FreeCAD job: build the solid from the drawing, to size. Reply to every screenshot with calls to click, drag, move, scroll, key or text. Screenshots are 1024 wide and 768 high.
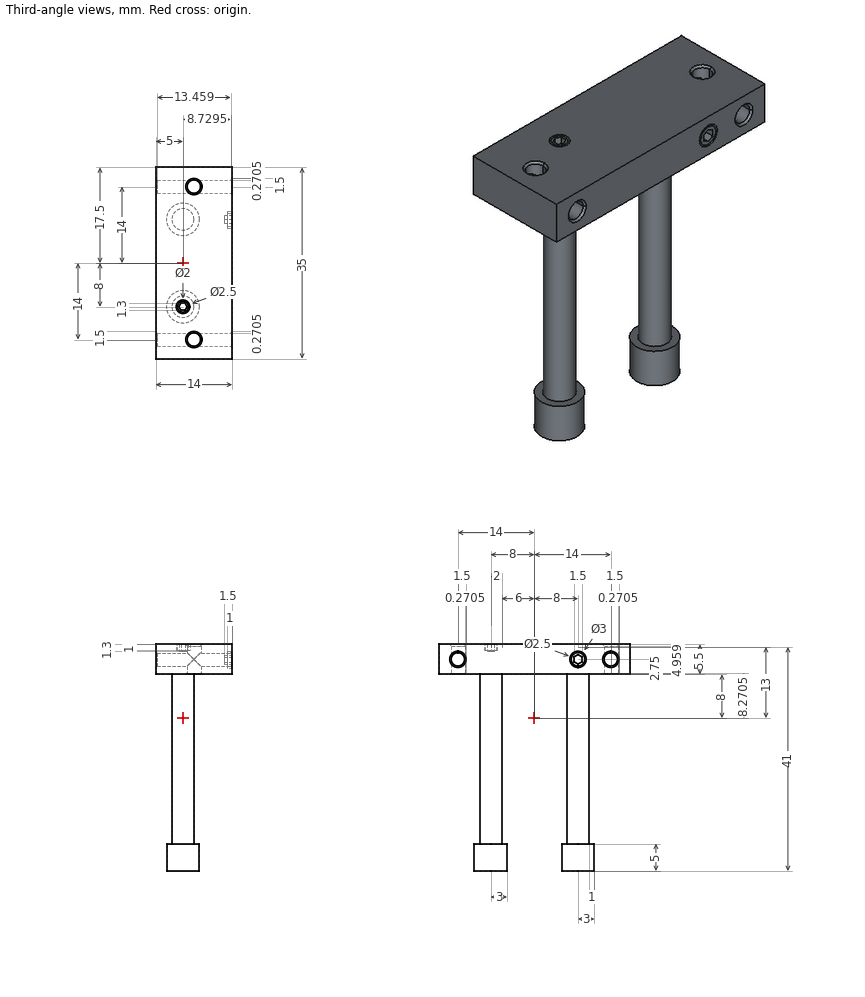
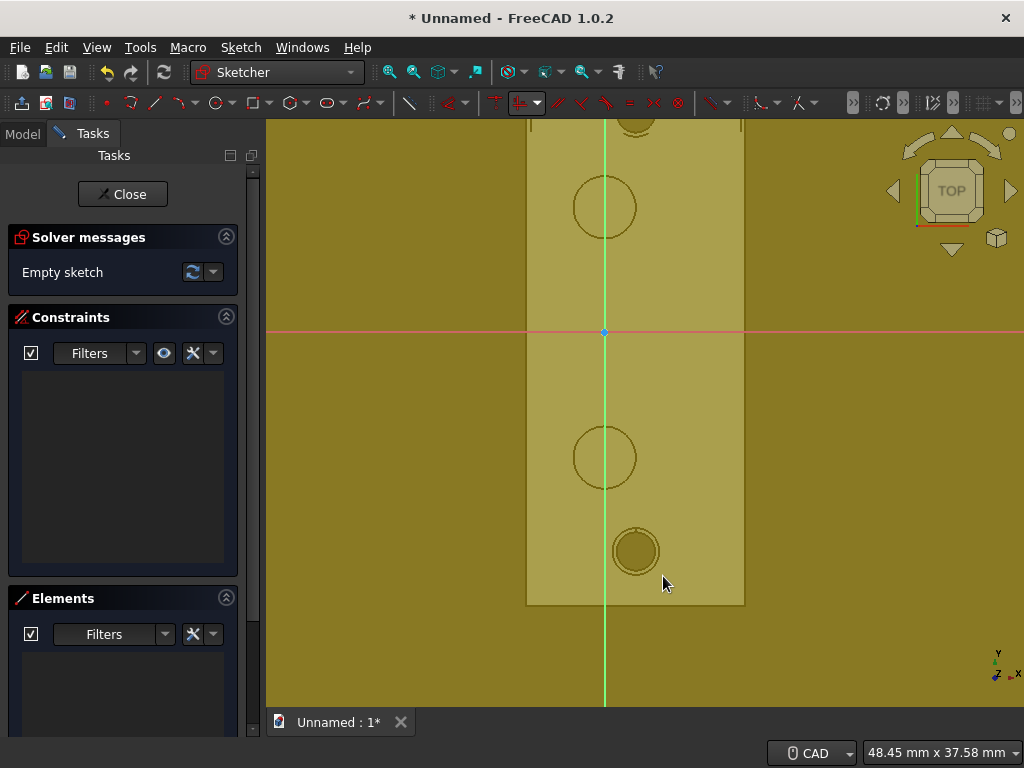
click(132, 104)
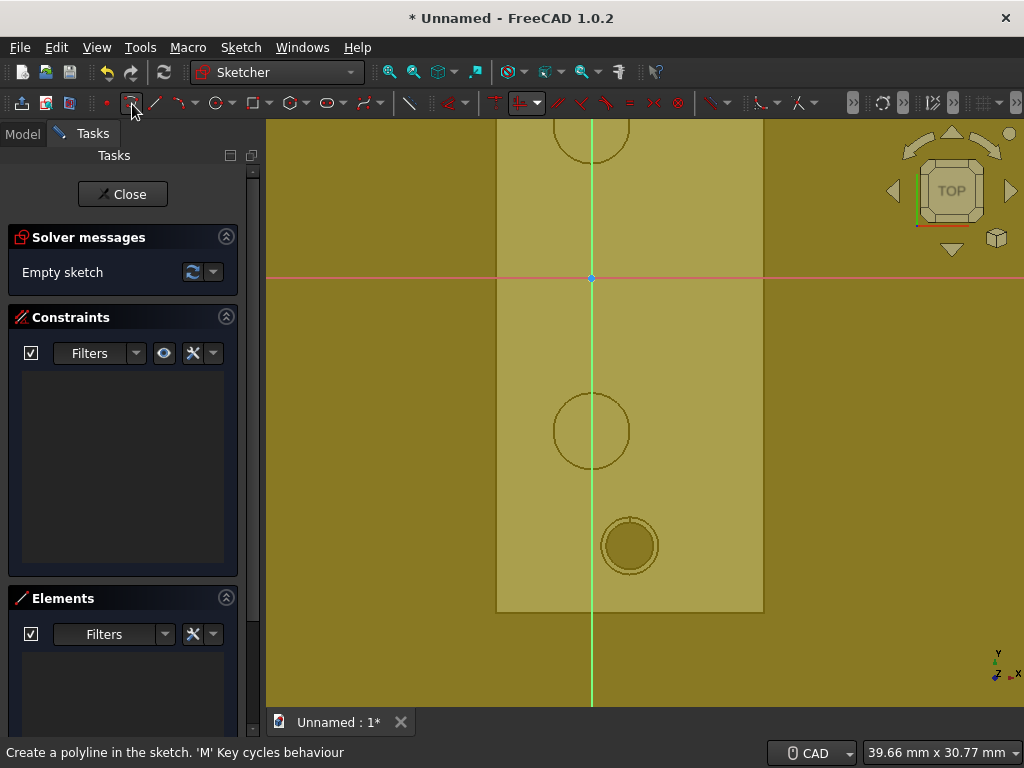
click(496, 517)
click(496, 546)
click(764, 546)
click(764, 517)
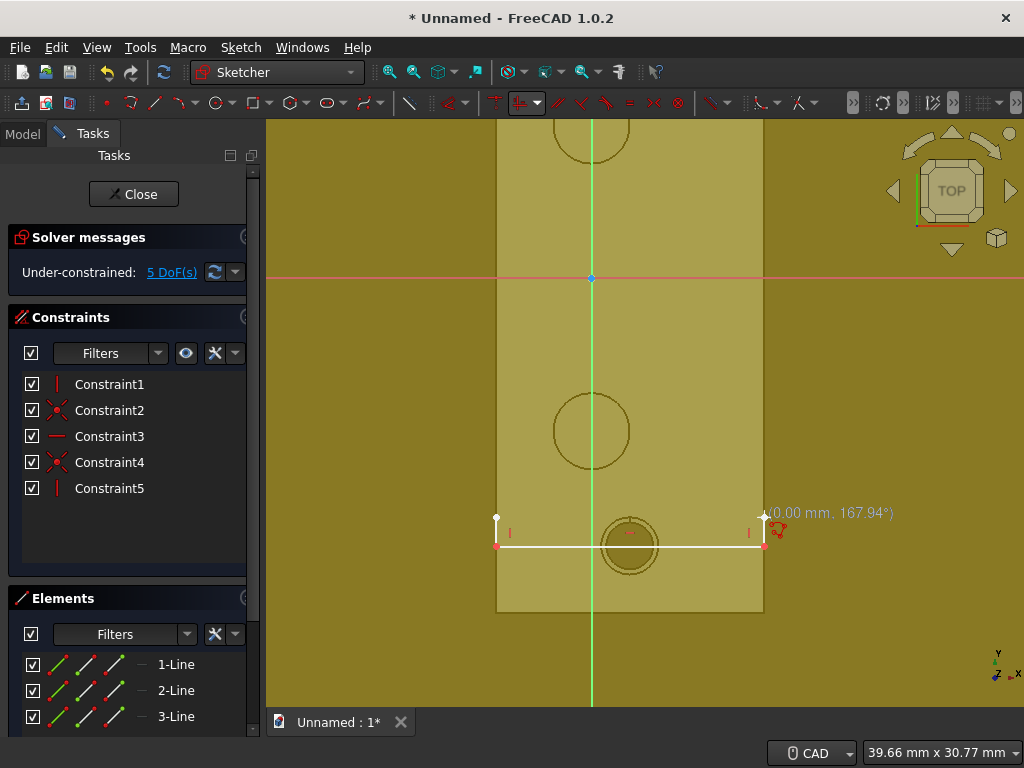
scroll(758, 522, up, 6)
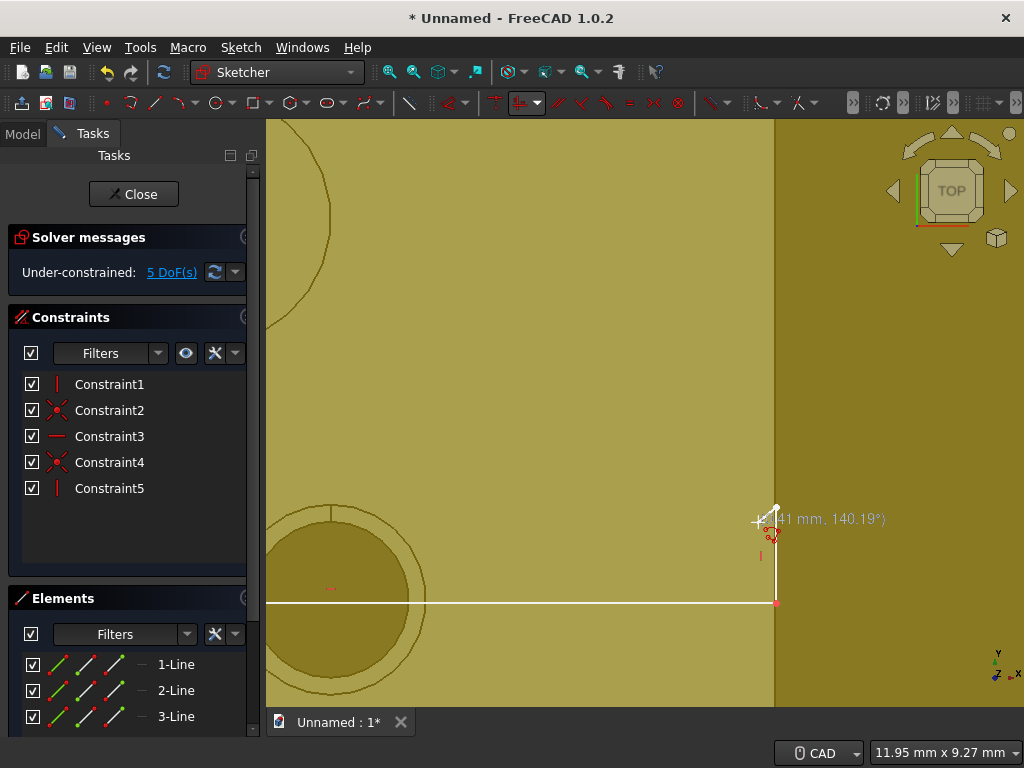
click(758, 522)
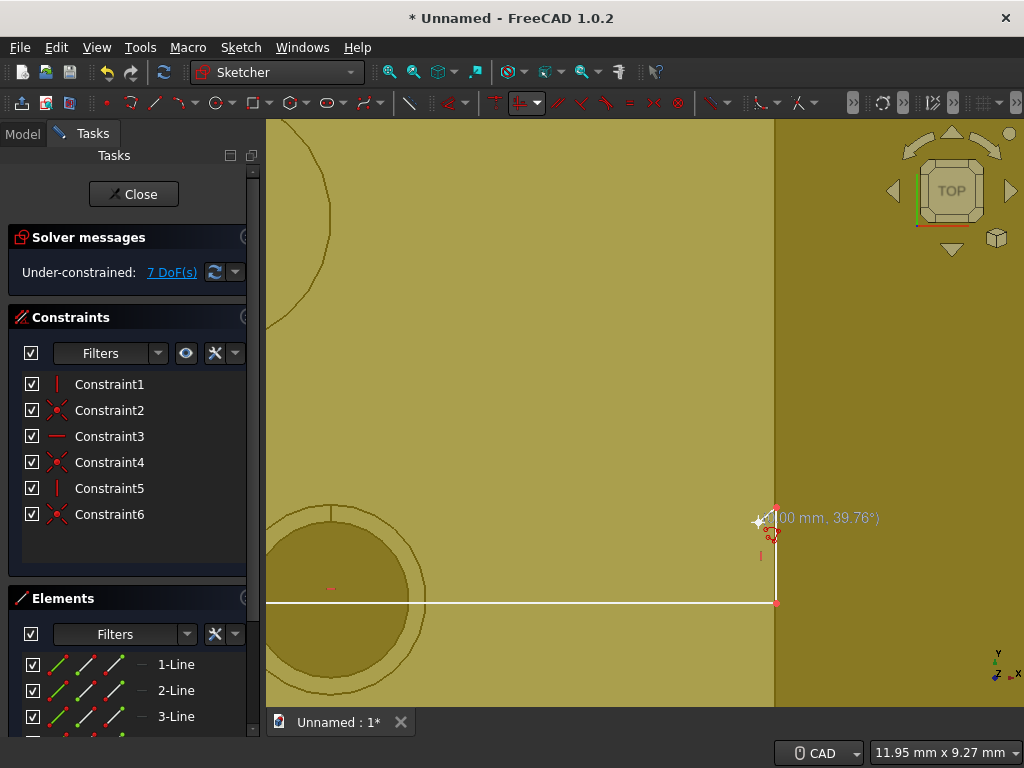
scroll(759, 524, down, 6)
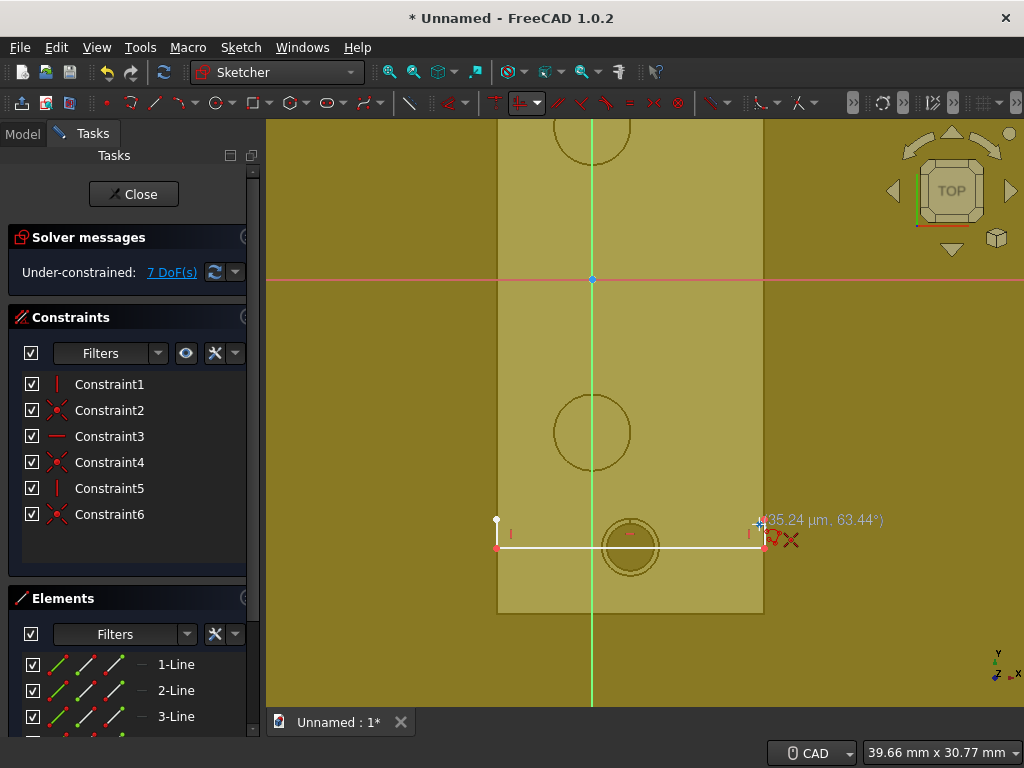
scroll(502, 524, up, 6)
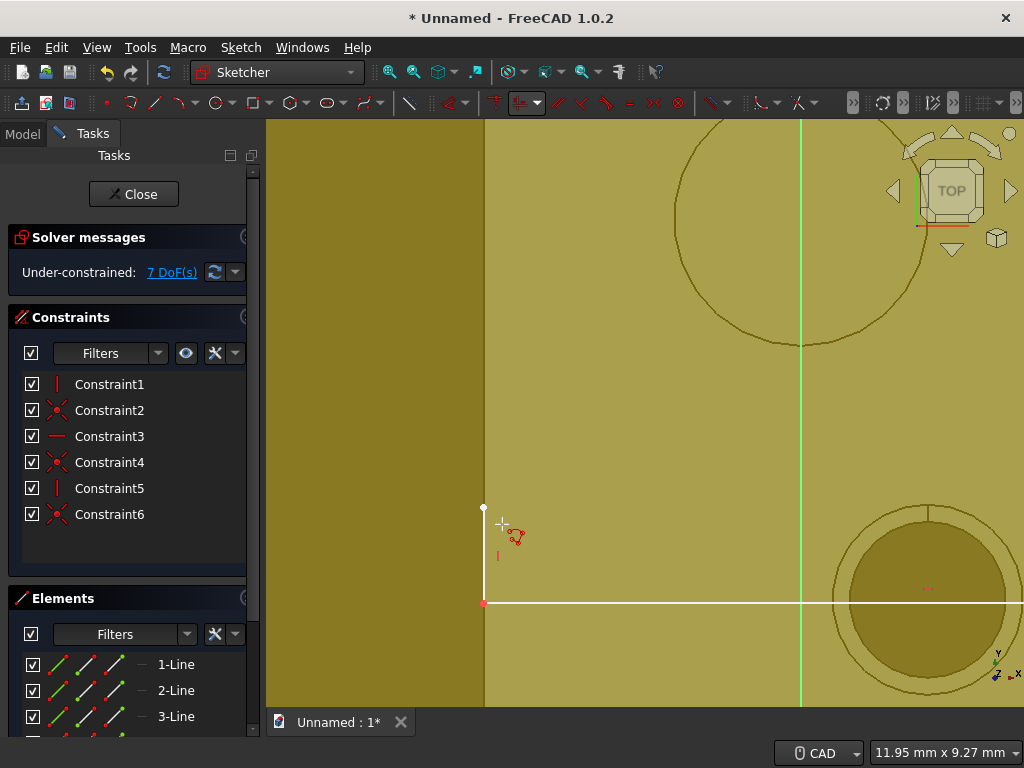
click(501, 522)
click(484, 507)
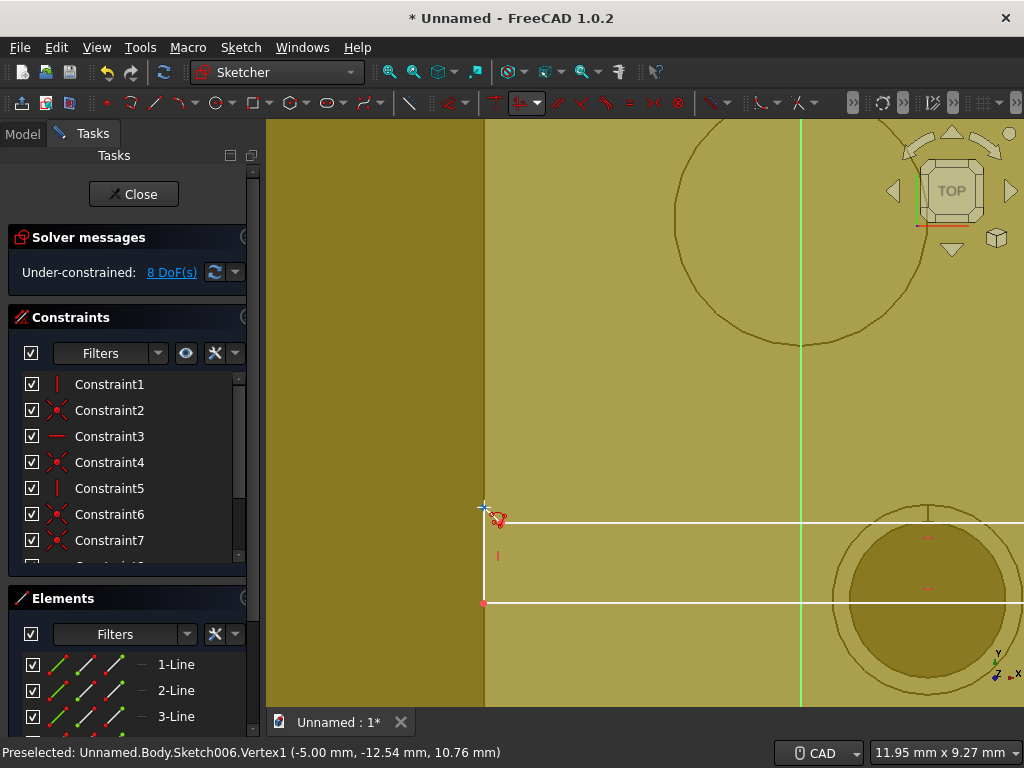
click(156, 104)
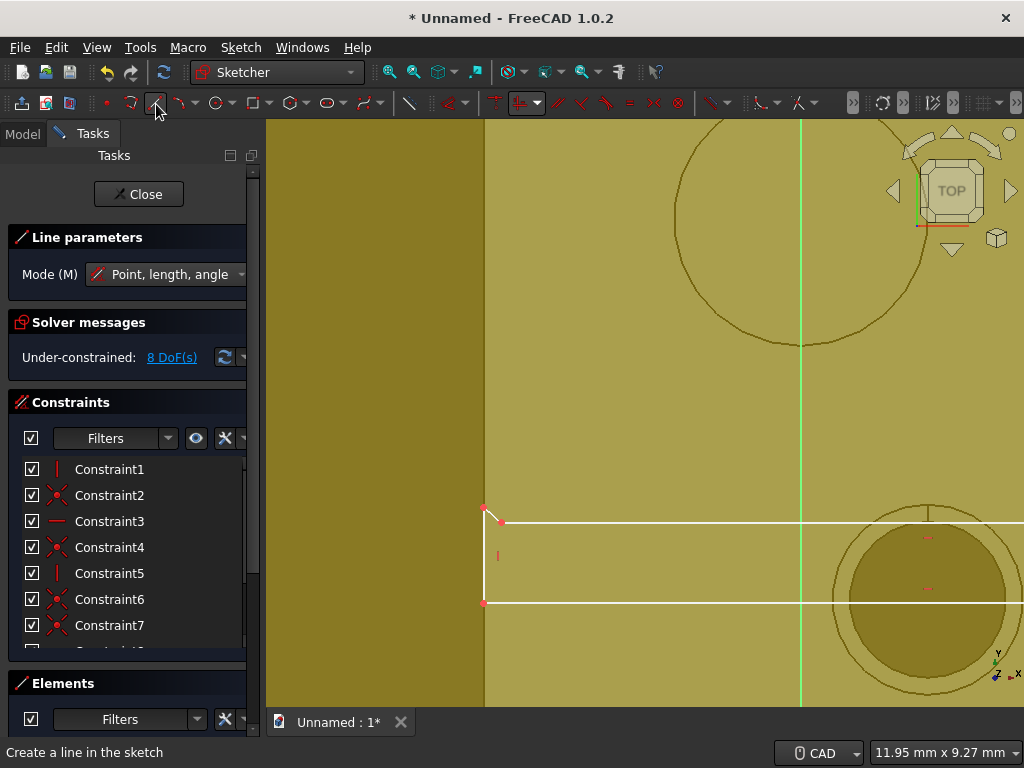
click(395, 600)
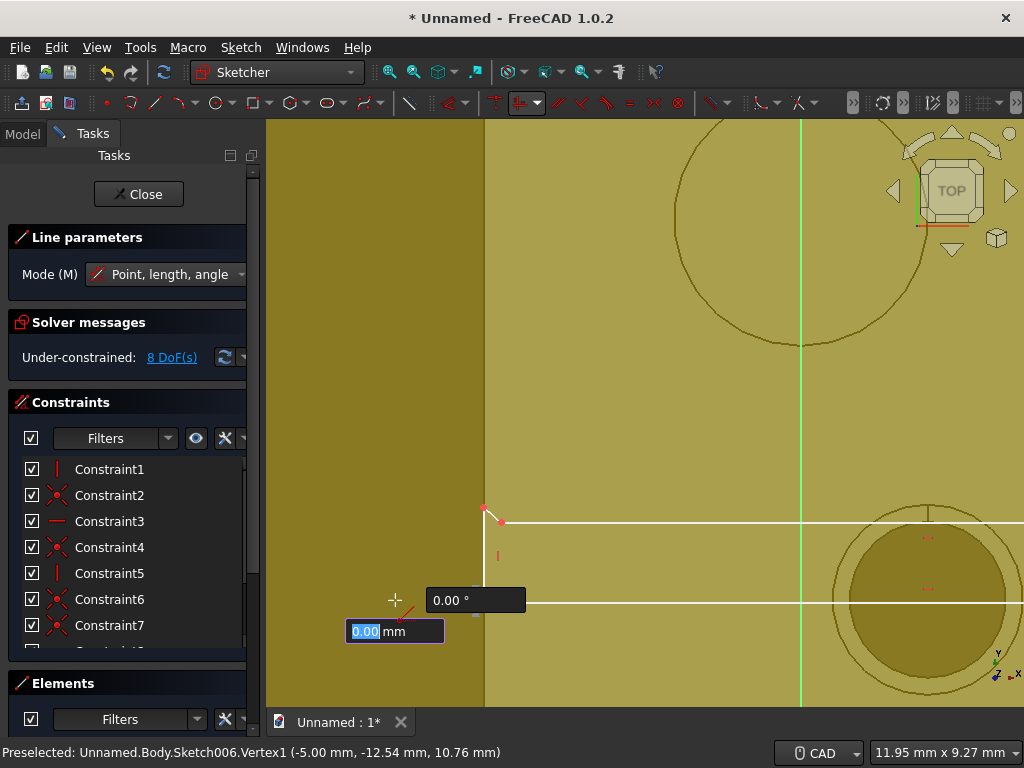
scroll(502, 524, down, 6)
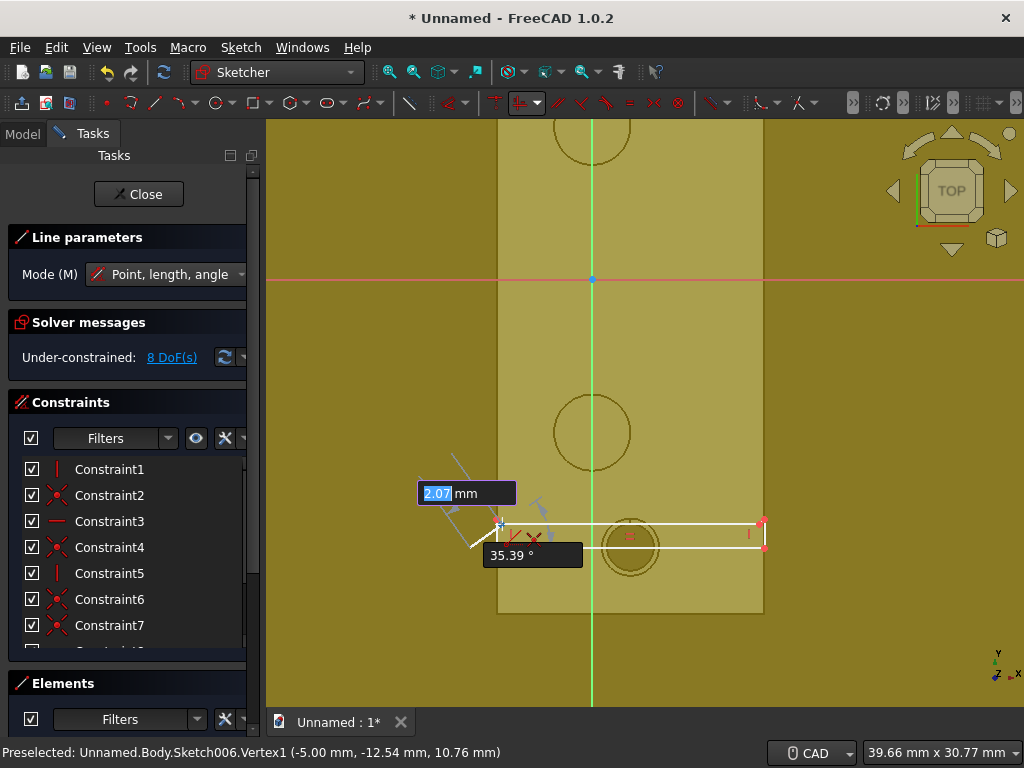
click(390, 547)
key(Escape)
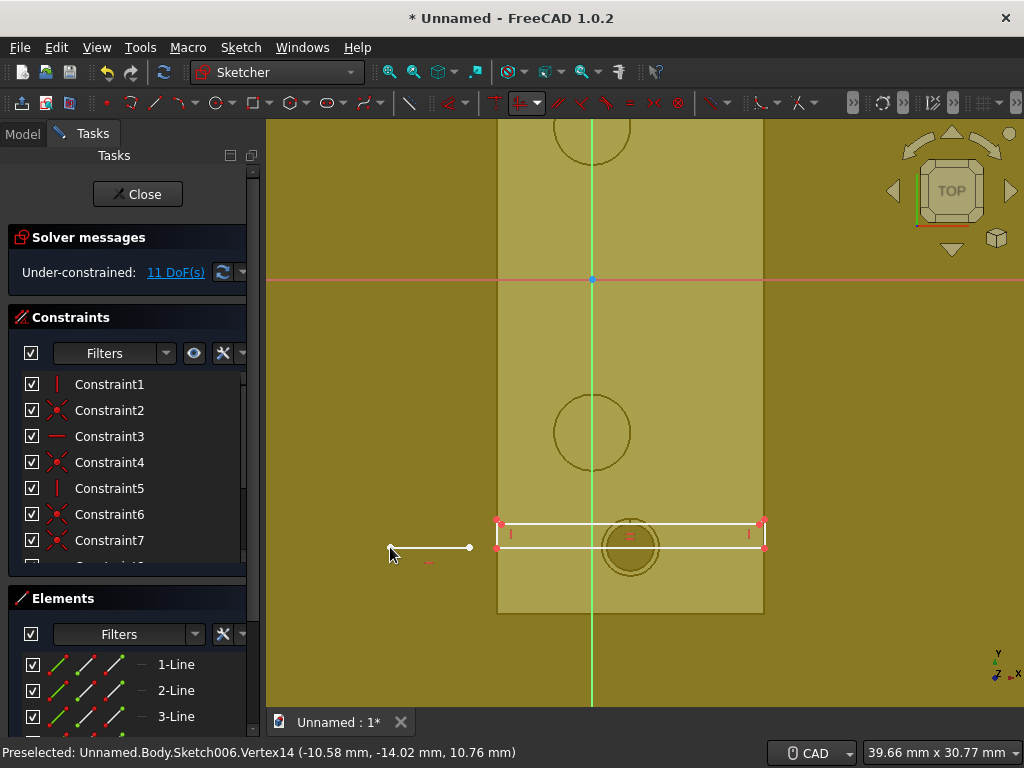
click(446, 548)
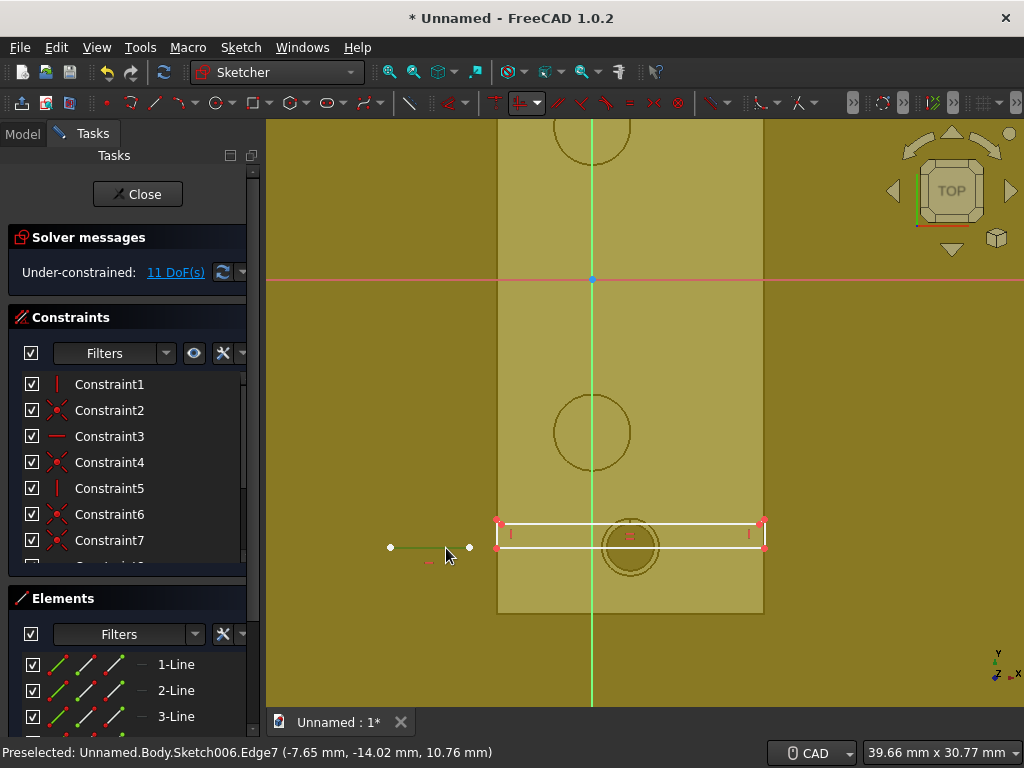
click(410, 104)